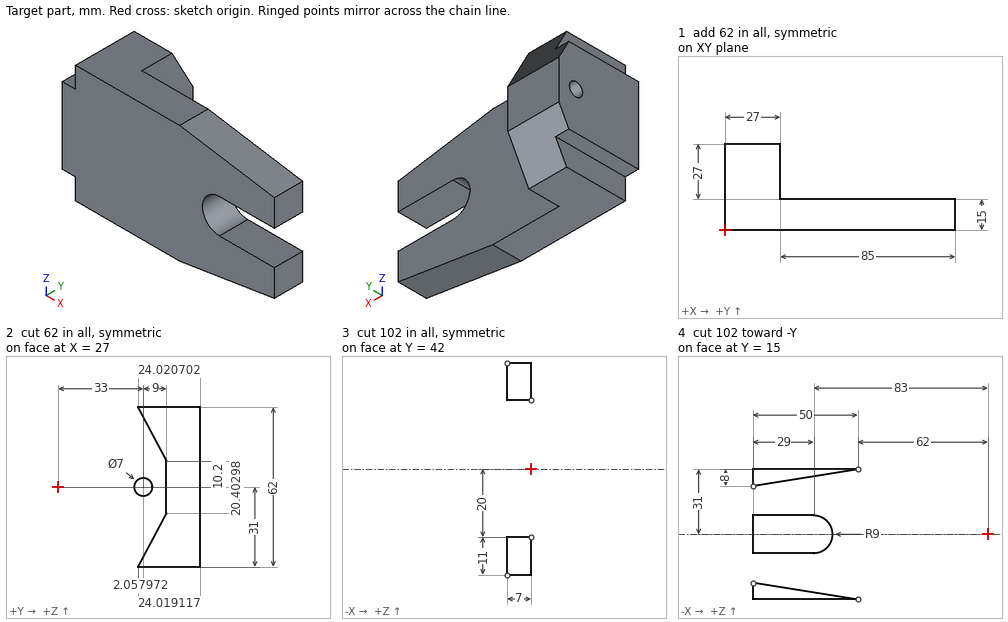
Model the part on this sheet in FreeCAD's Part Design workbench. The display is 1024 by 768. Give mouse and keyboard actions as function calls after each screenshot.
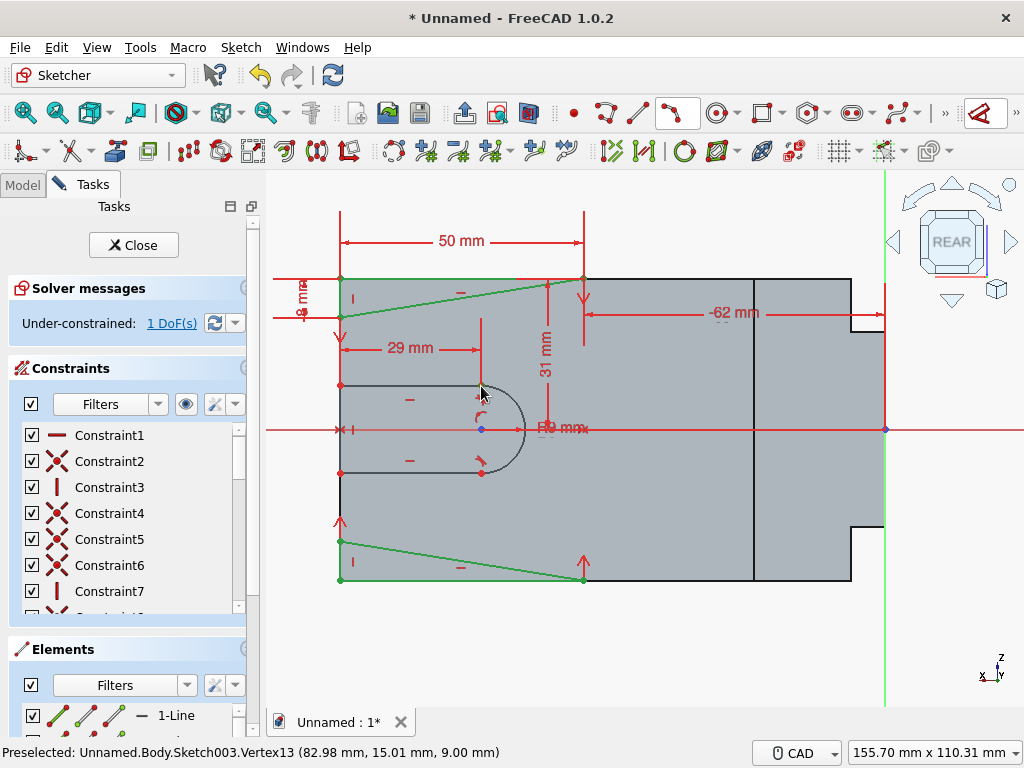
click(1002, 114)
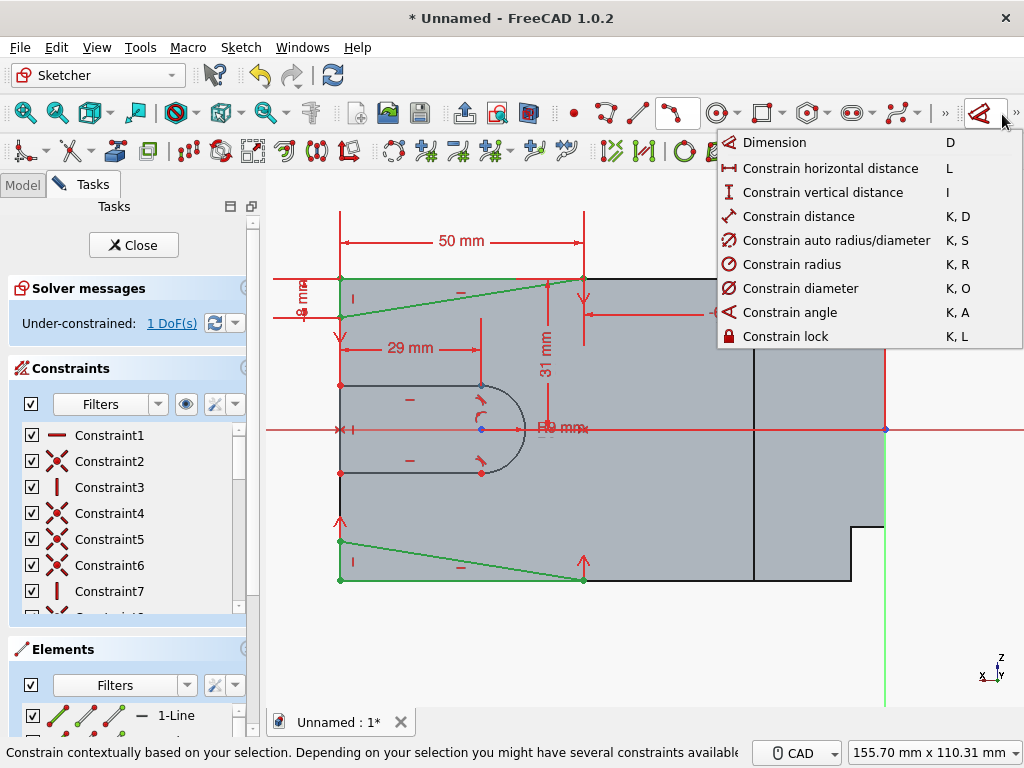
click(870, 168)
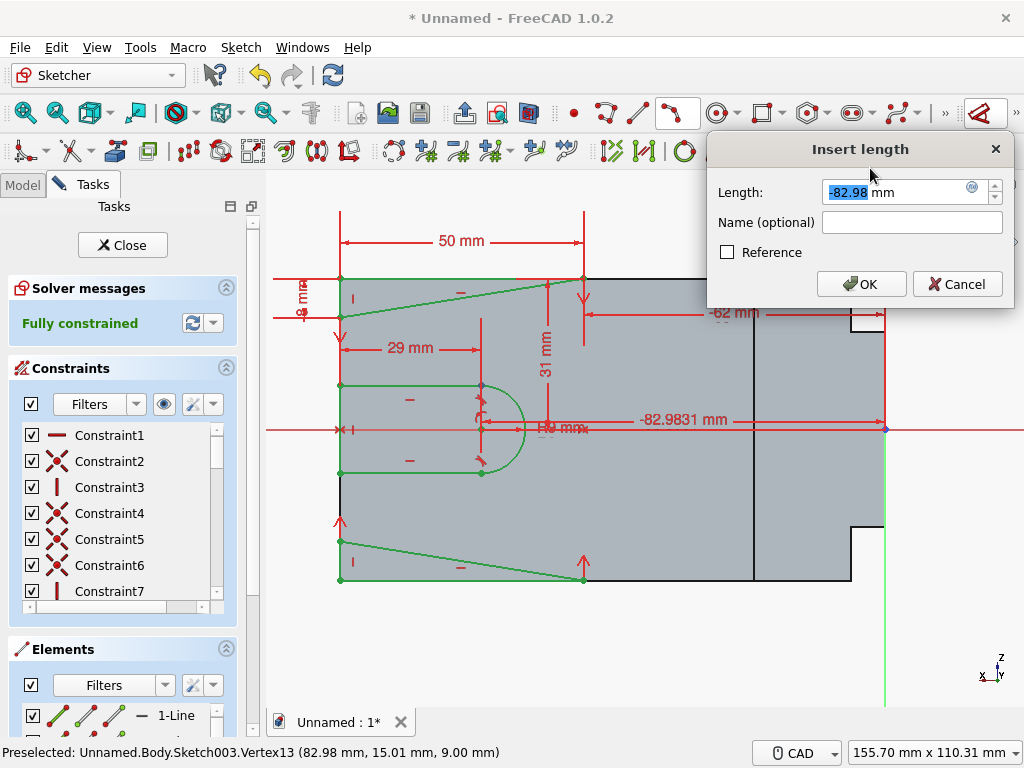
text(-83)
key(Return)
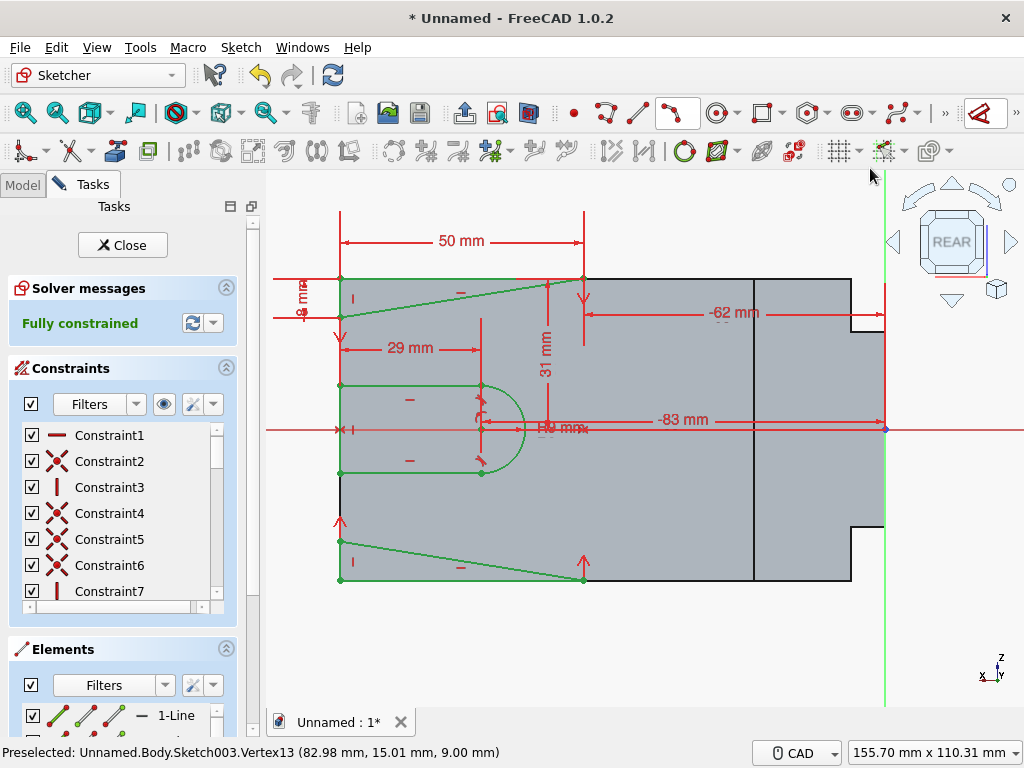
click(123, 245)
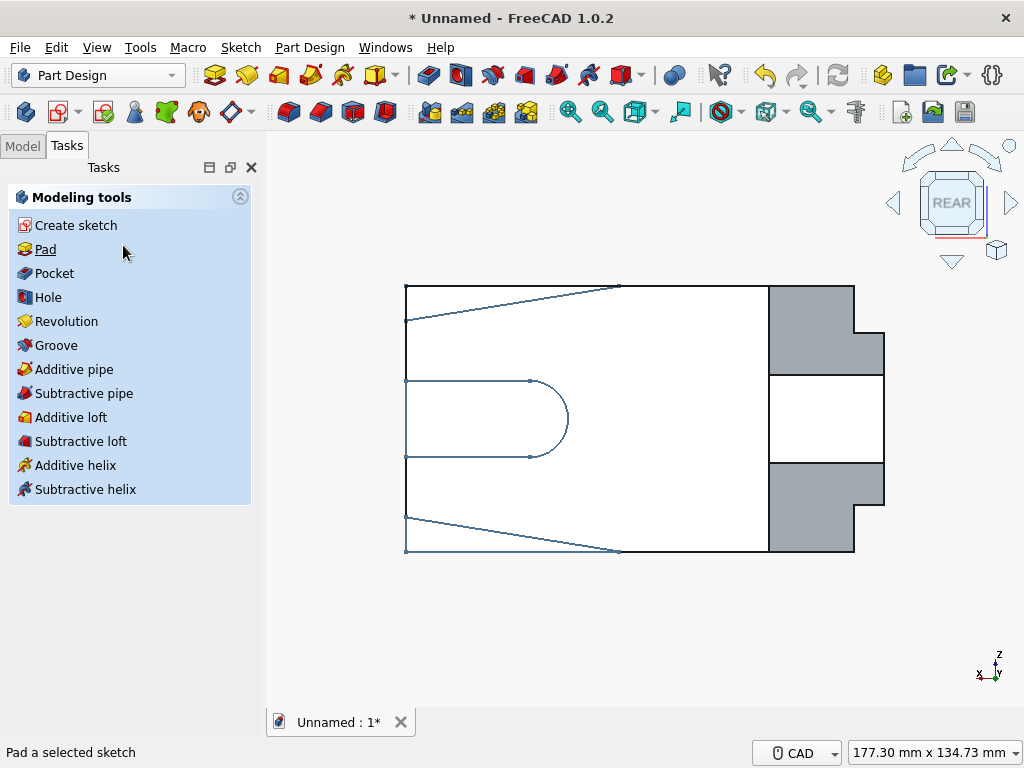
click(430, 76)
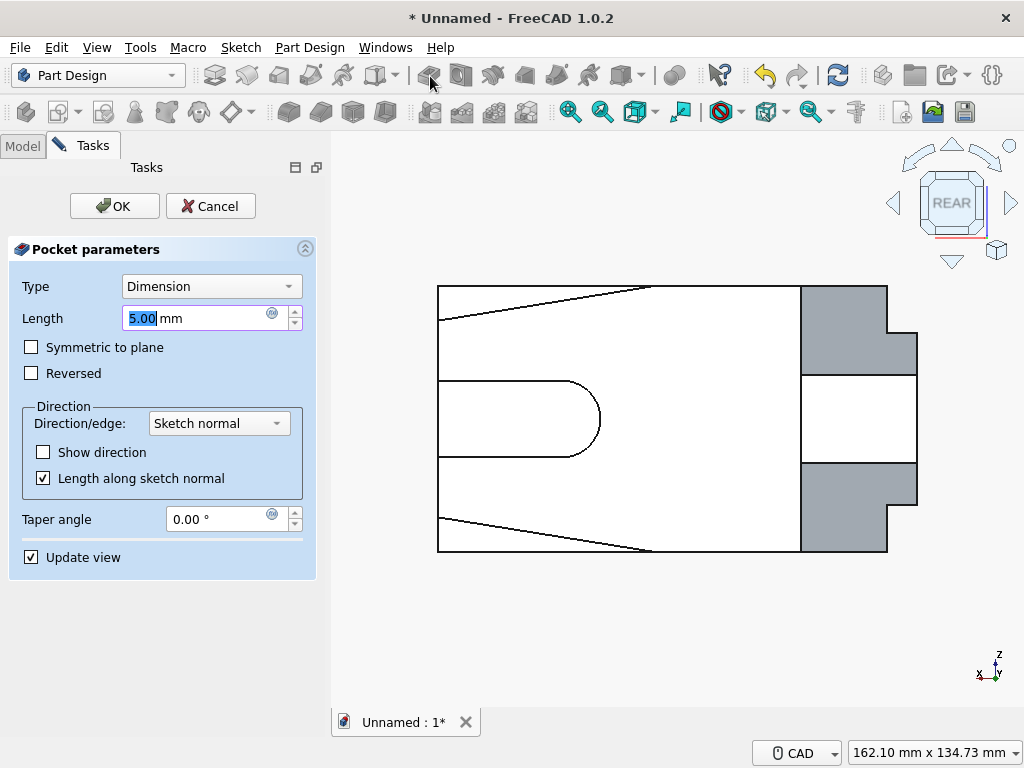
text(102)
key(Tab)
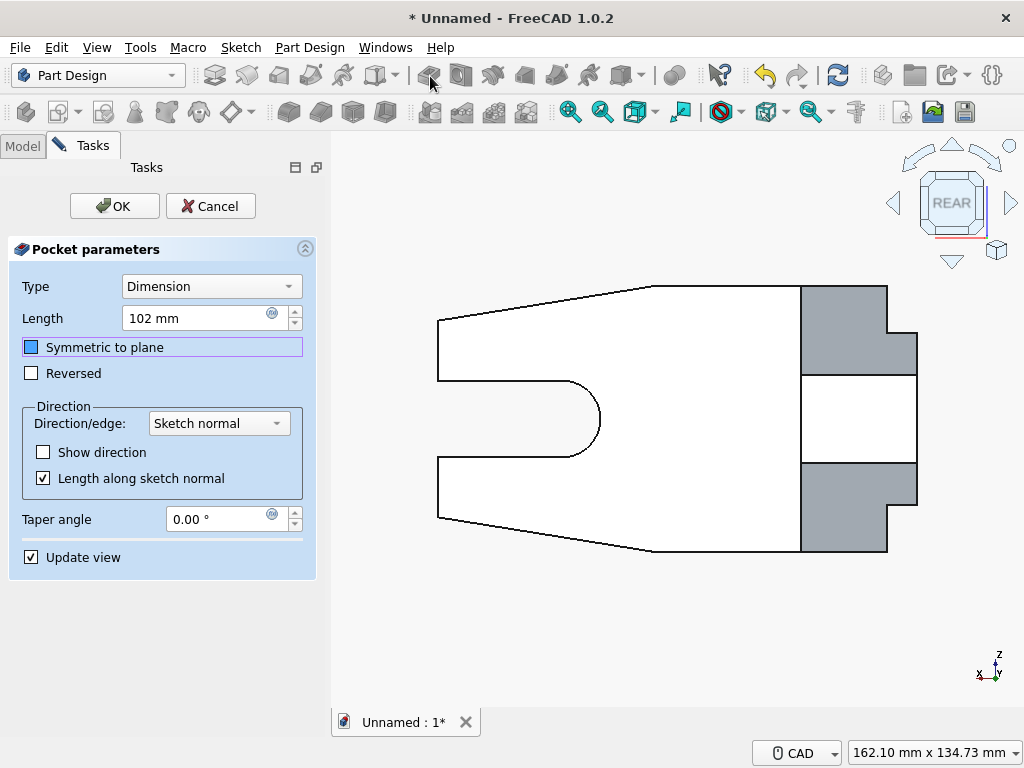
click(115, 206)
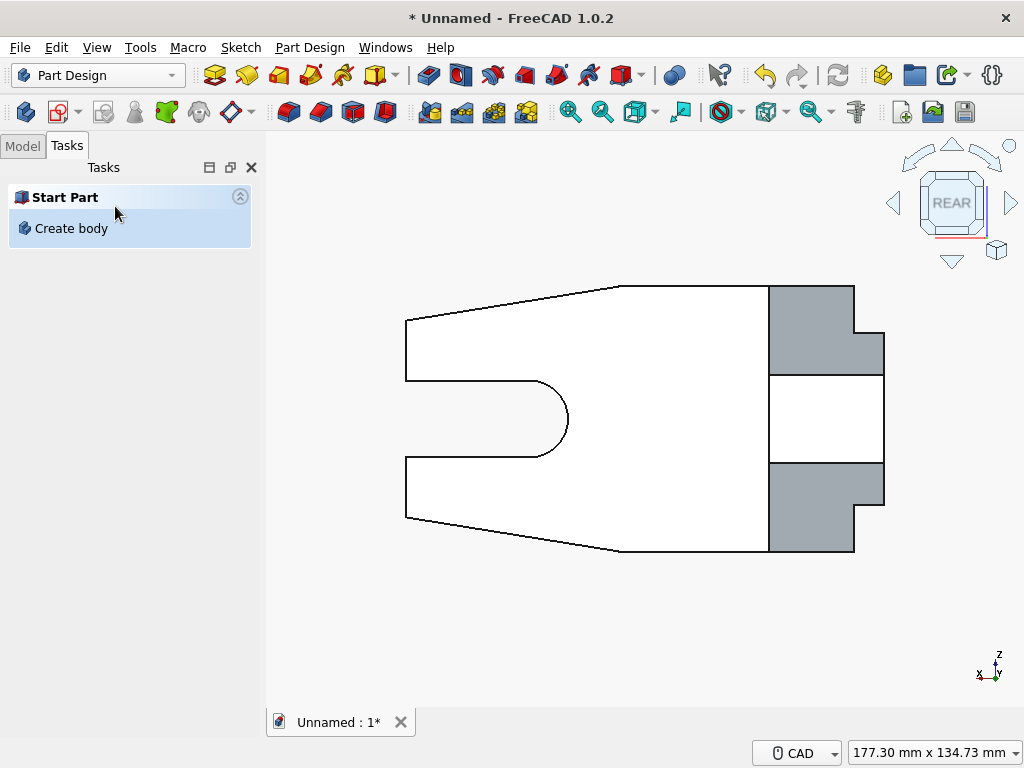
key(0)